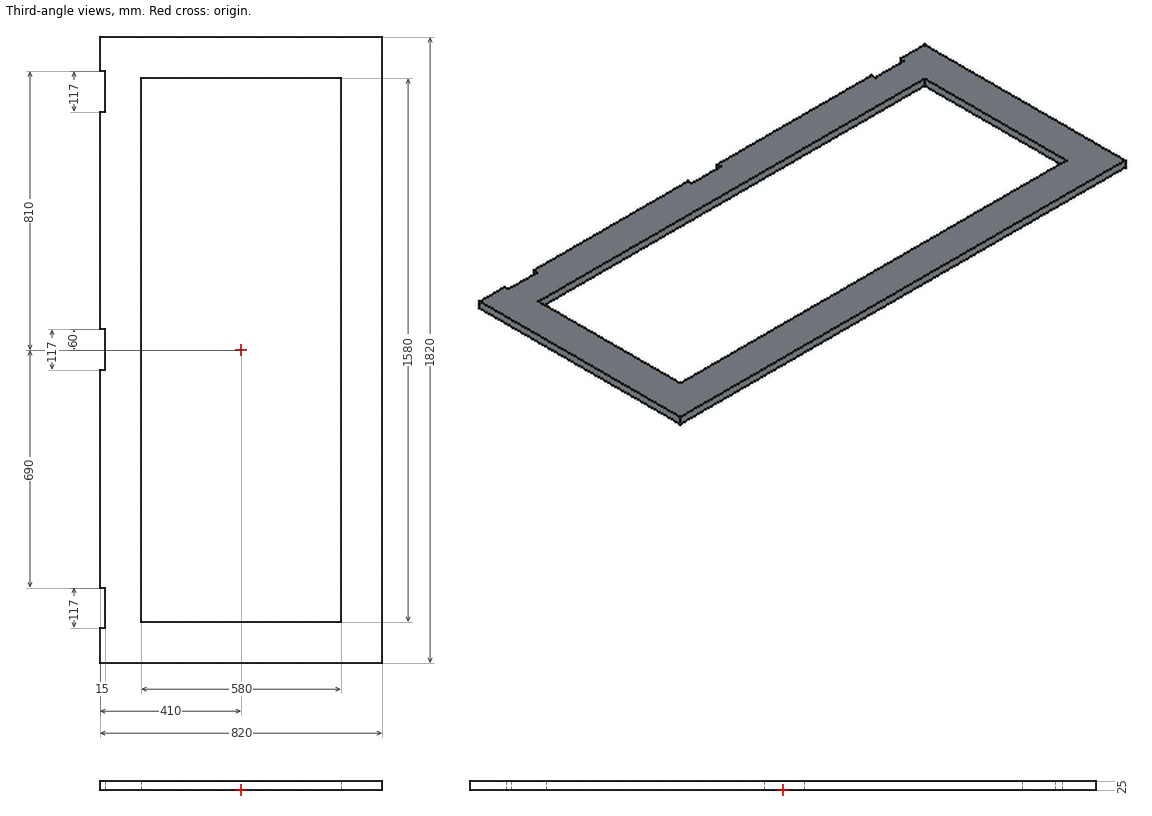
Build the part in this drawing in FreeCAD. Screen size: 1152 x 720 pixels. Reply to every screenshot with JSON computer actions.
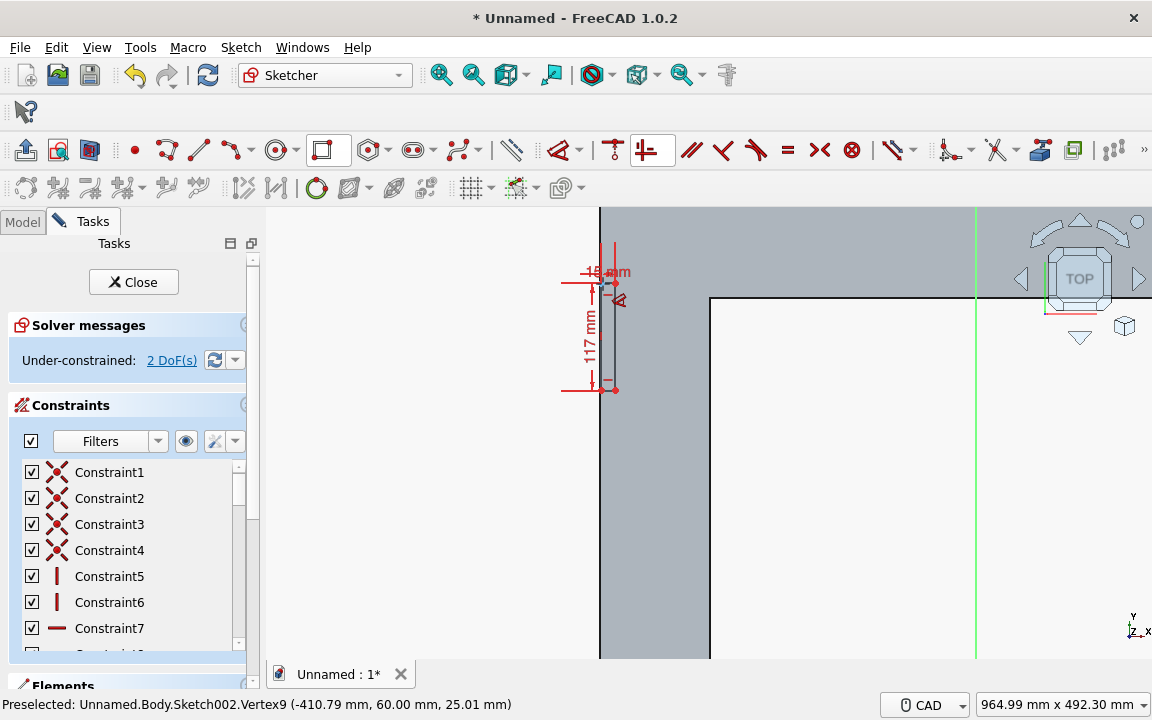
{"action": "left_click", "coordinate": [601, 283]}
{"action": "left_click", "coordinate": [789, 249]}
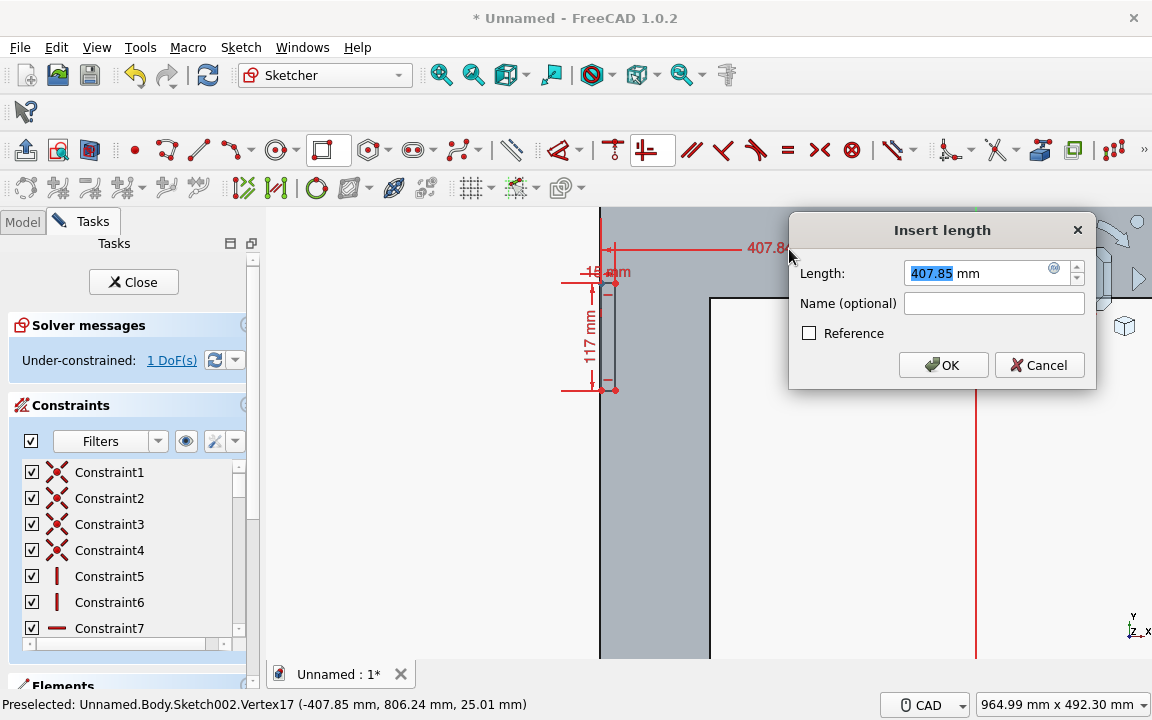
{"action": "type", "text": "410"}
{"action": "key", "text": "Return"}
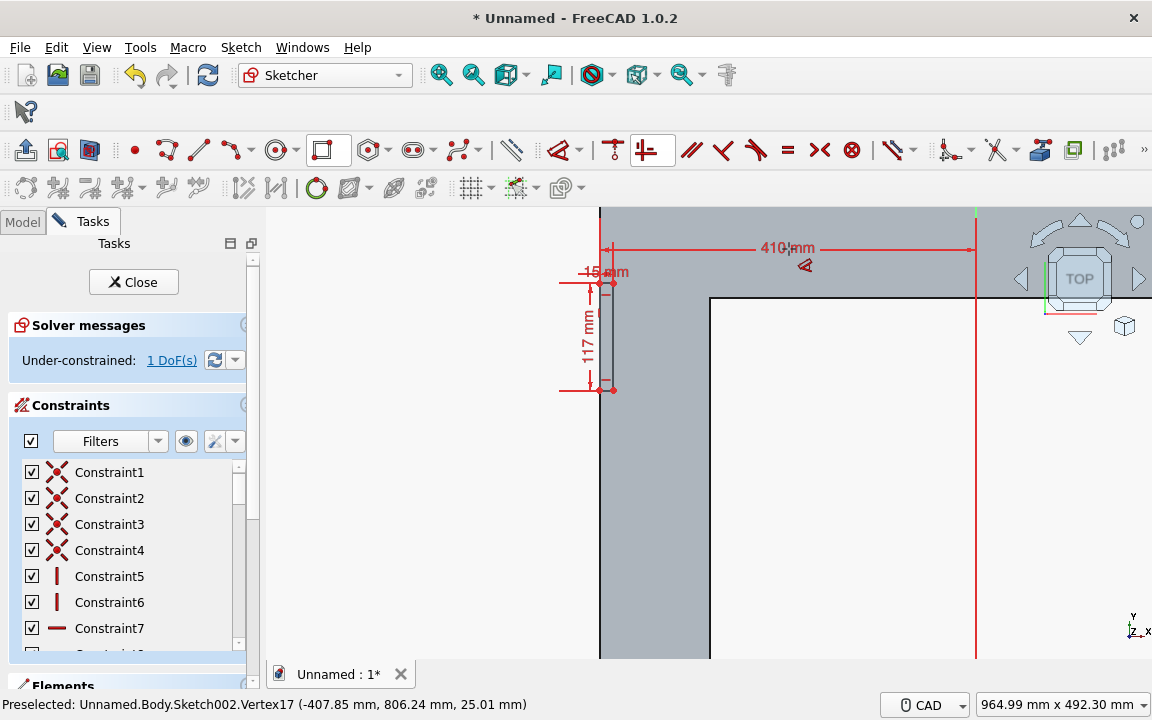
{"action": "left_click", "coordinate": [600, 283]}
{"action": "left_click", "coordinate": [566, 457]}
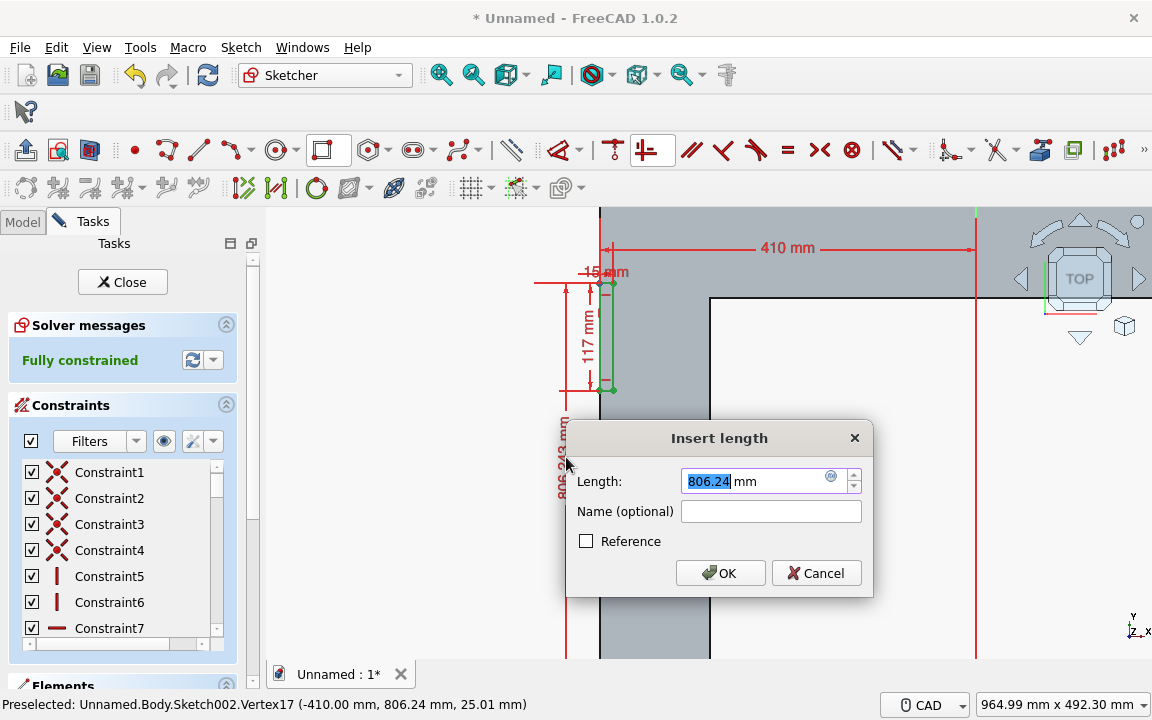
{"action": "type", "text": "810"}
{"action": "key", "text": "Return"}
{"action": "key", "text": "Escape"}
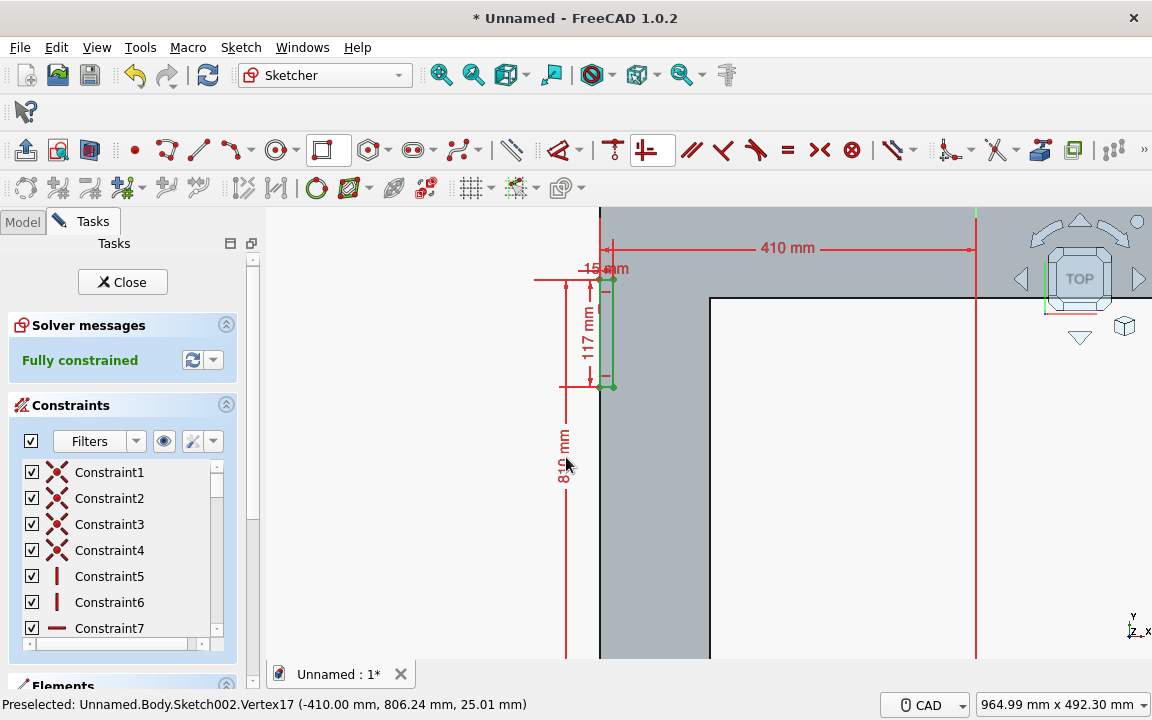
{"action": "left_click", "coordinate": [123, 282]}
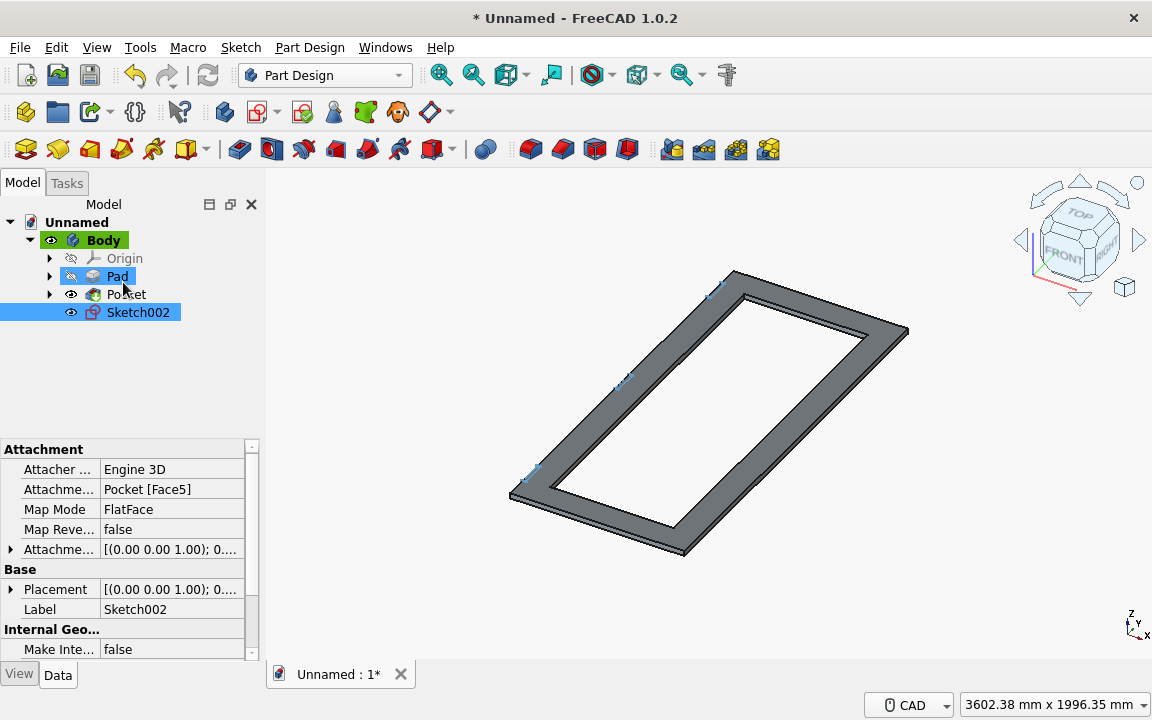
{"action": "left_click", "coordinate": [240, 150]}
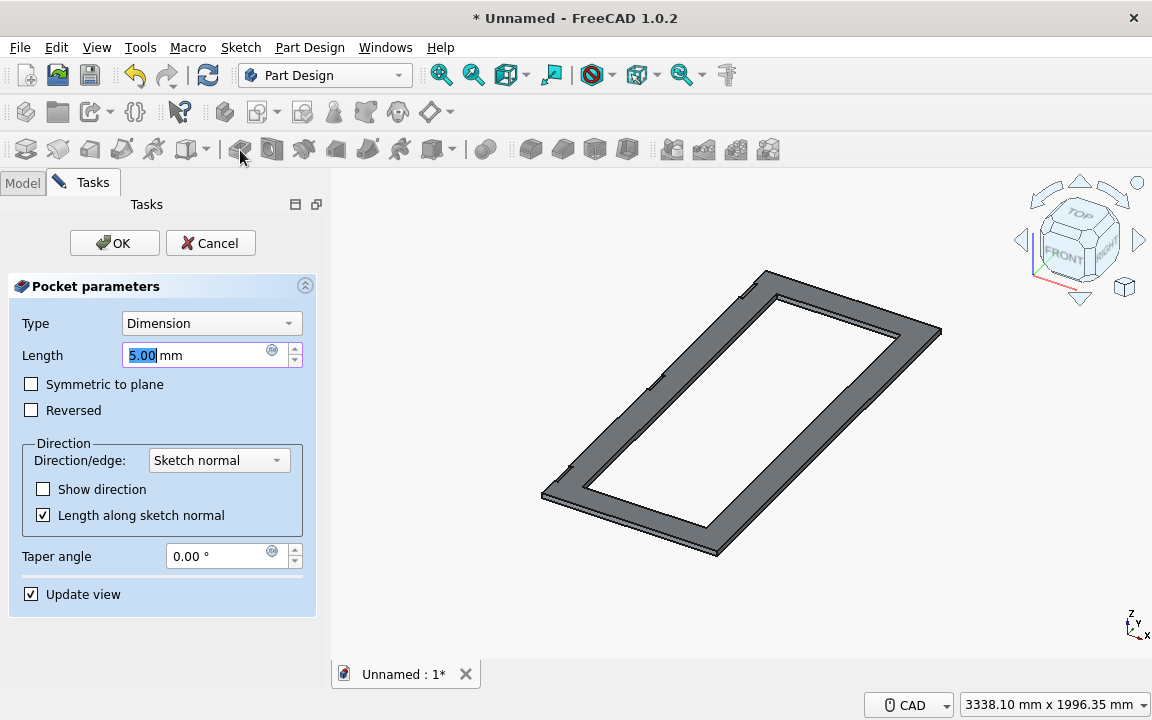
{"action": "left_click", "coordinate": [212, 324]}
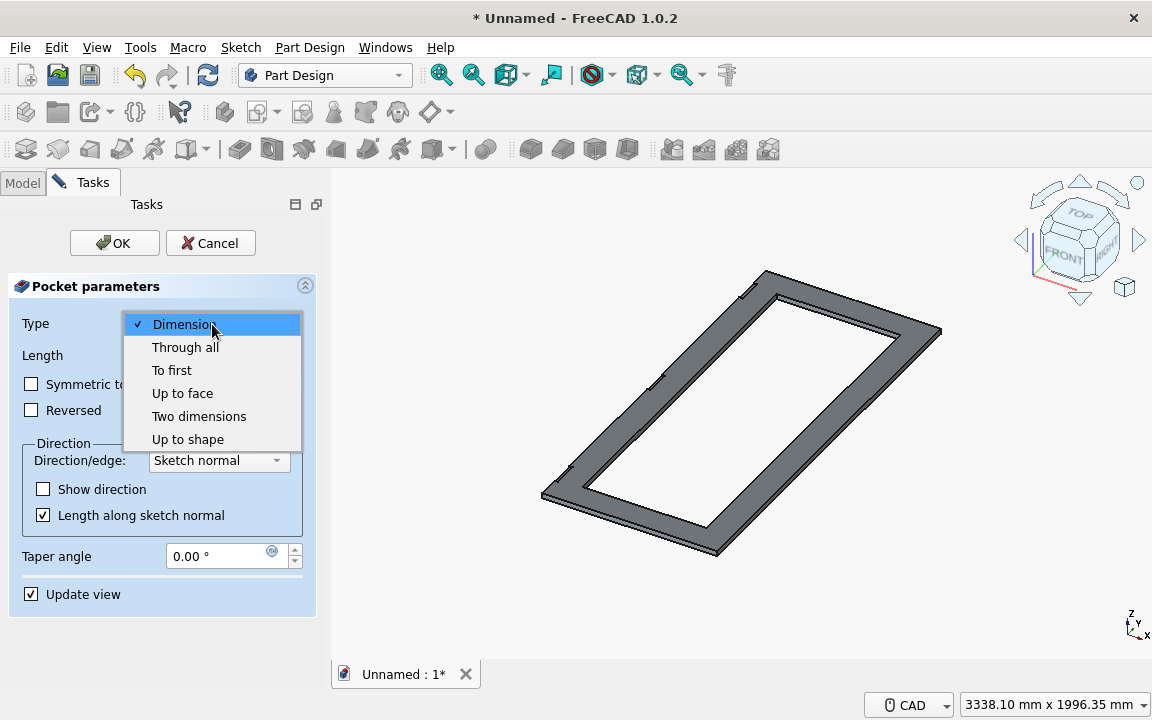
{"action": "left_click", "coordinate": [212, 348]}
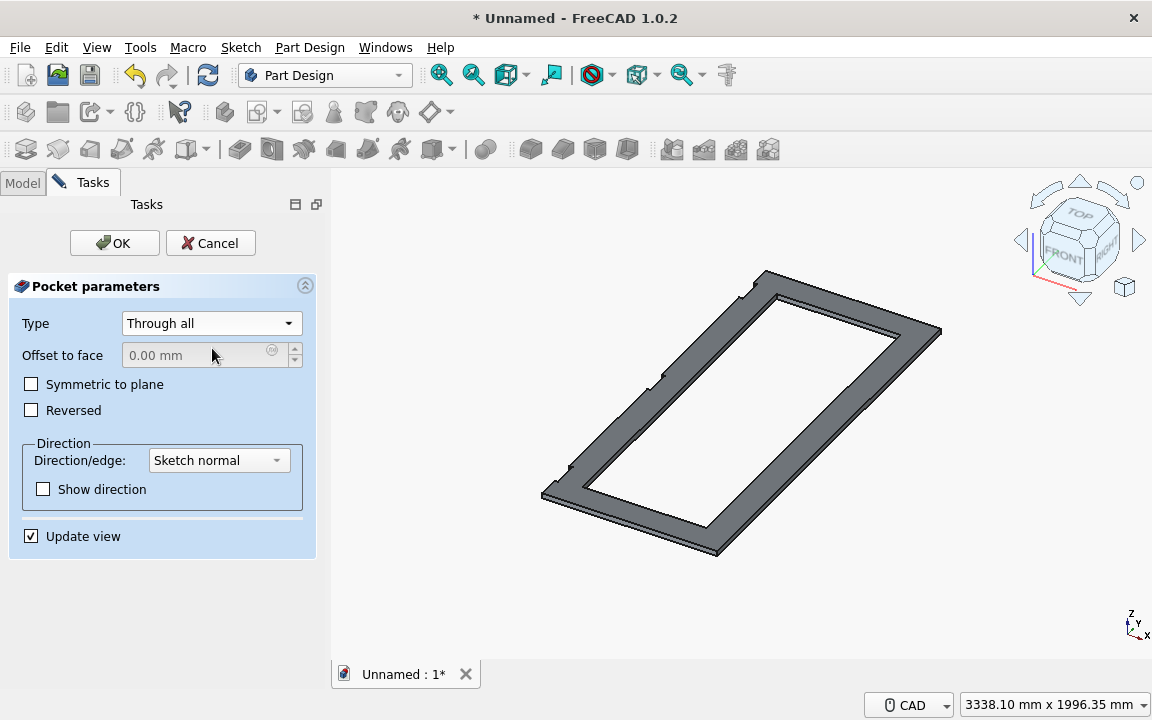
{"action": "left_click", "coordinate": [115, 243]}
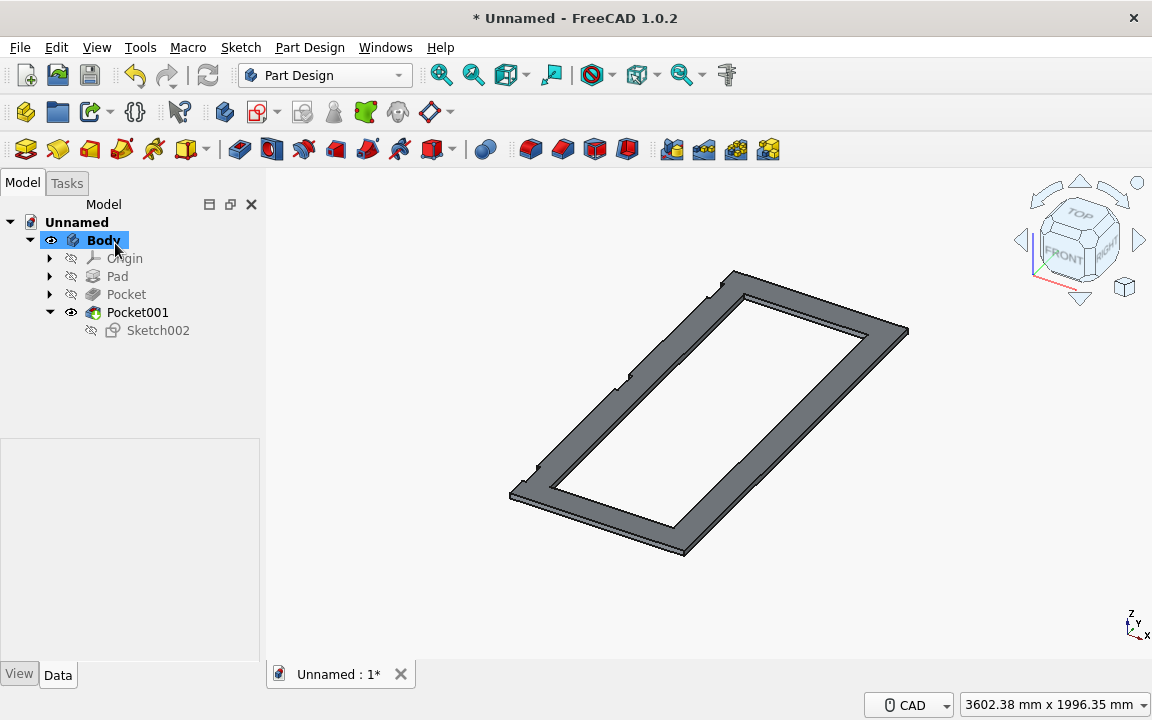
{"action": "key", "text": "0"}